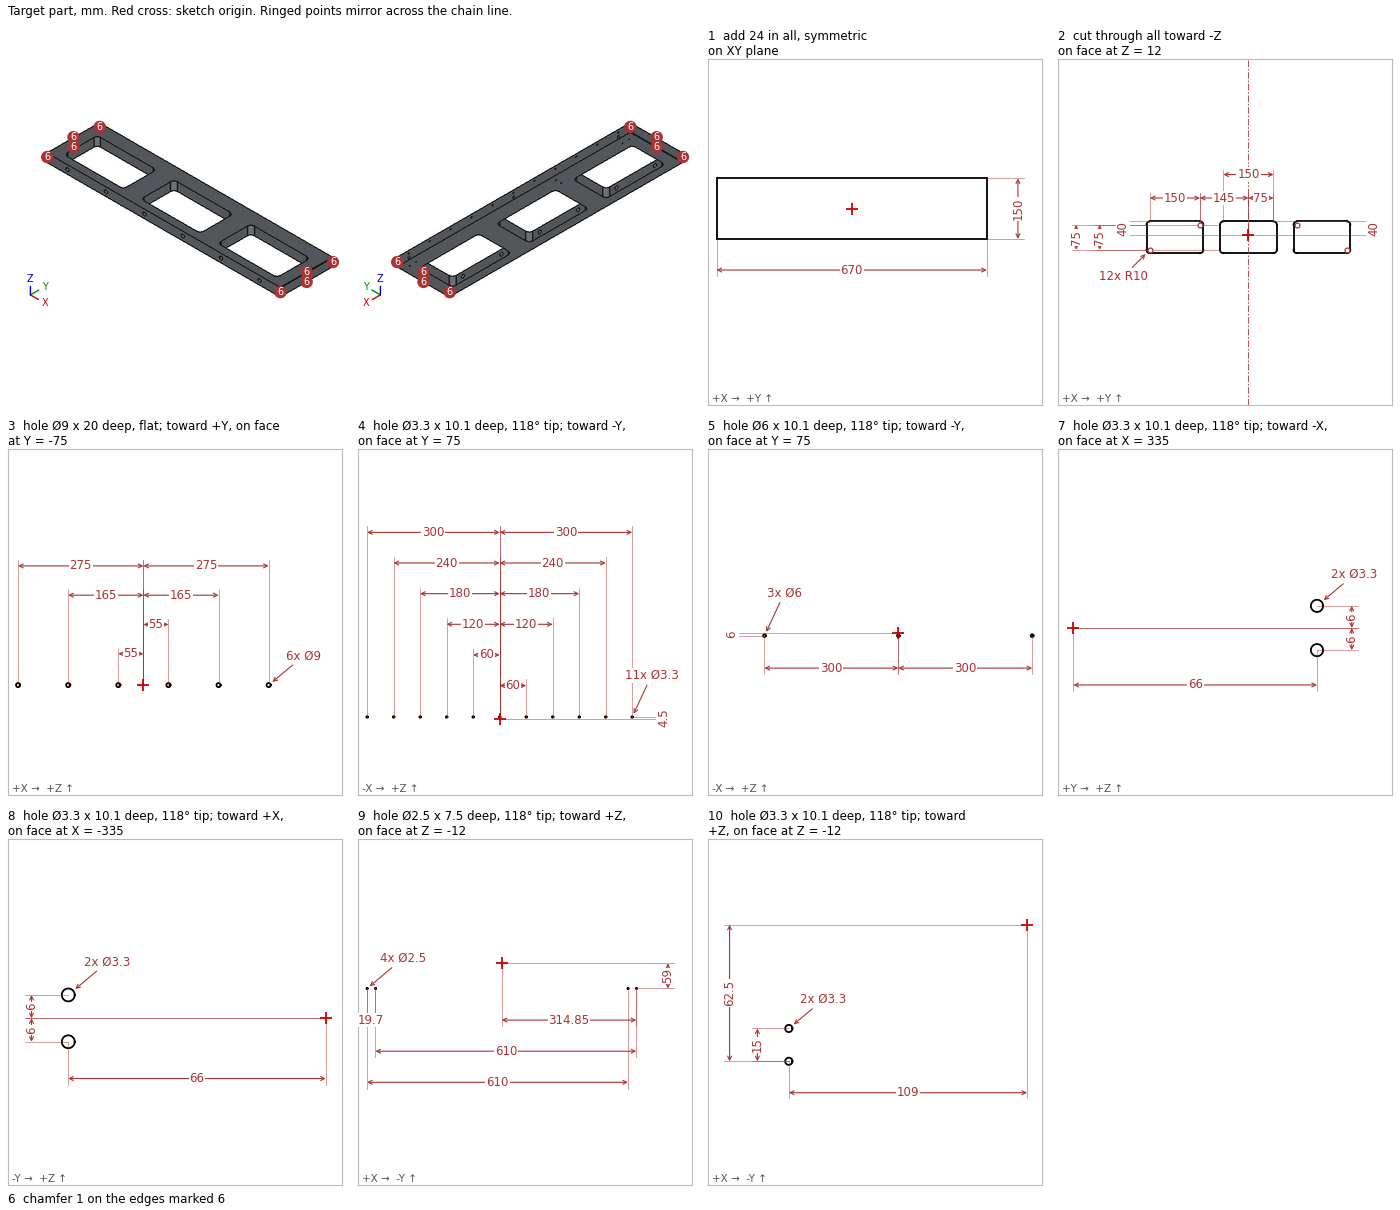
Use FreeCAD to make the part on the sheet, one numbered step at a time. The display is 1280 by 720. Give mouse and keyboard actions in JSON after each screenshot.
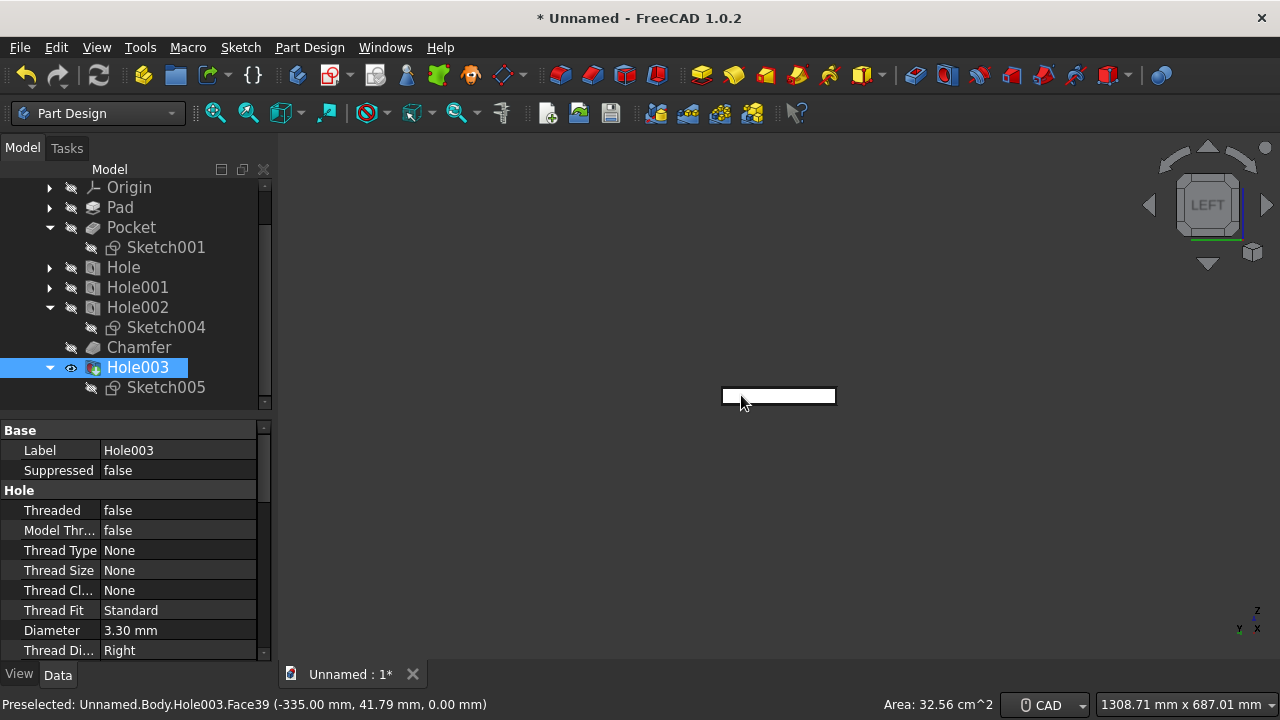
{"action": "left_click", "coordinate": [330, 76]}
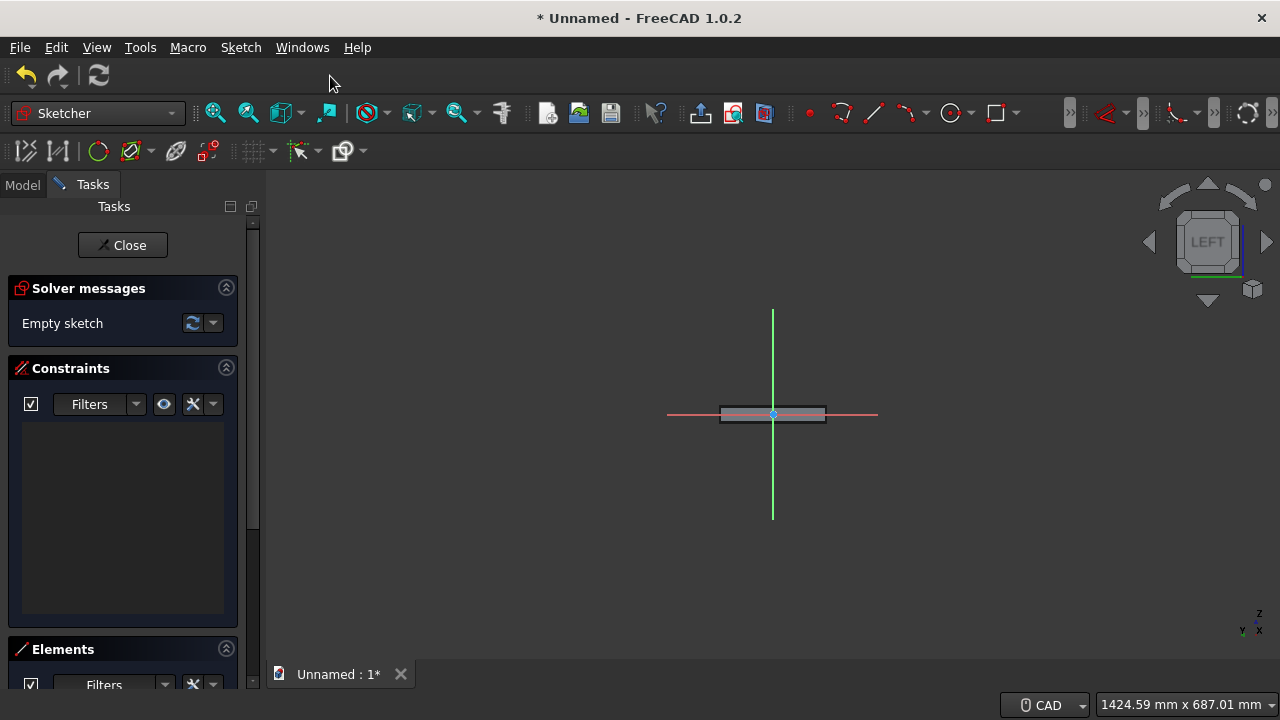
{"action": "scroll", "coordinate": [727, 414], "scroll_direction": "up", "scroll_amount": 15}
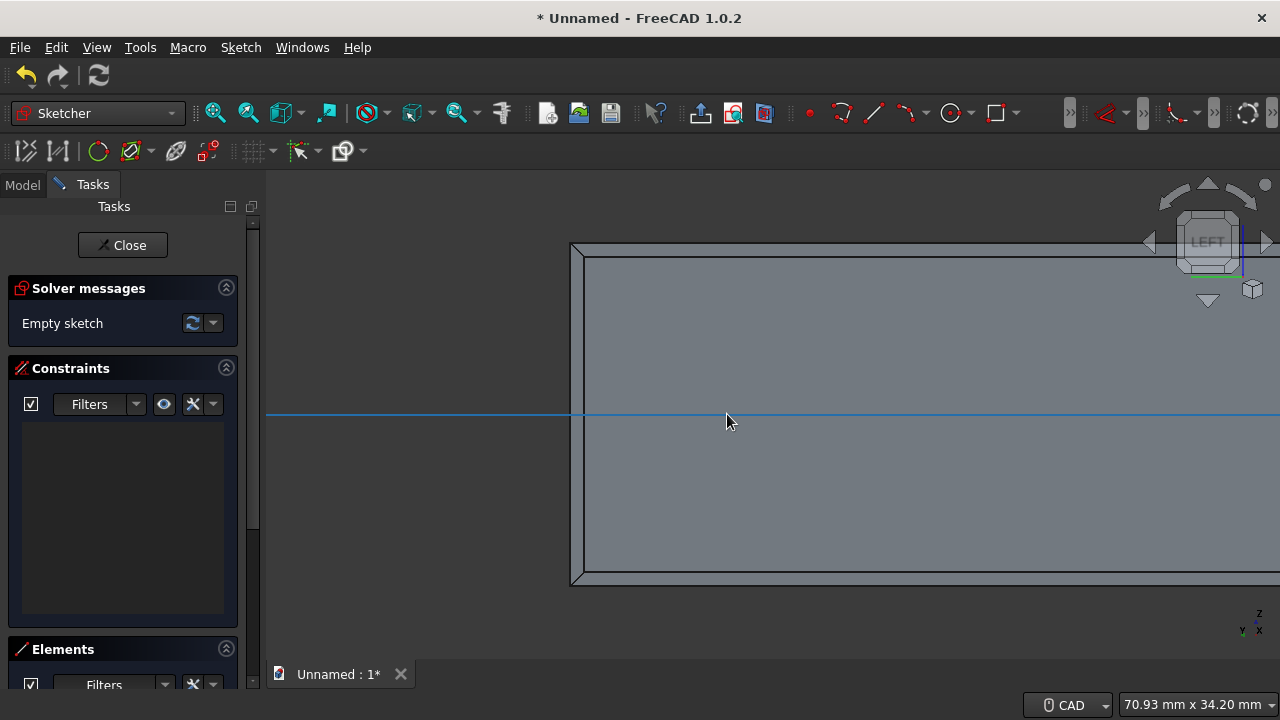
{"action": "scroll", "coordinate": [687, 414], "scroll_direction": "up", "scroll_amount": 2}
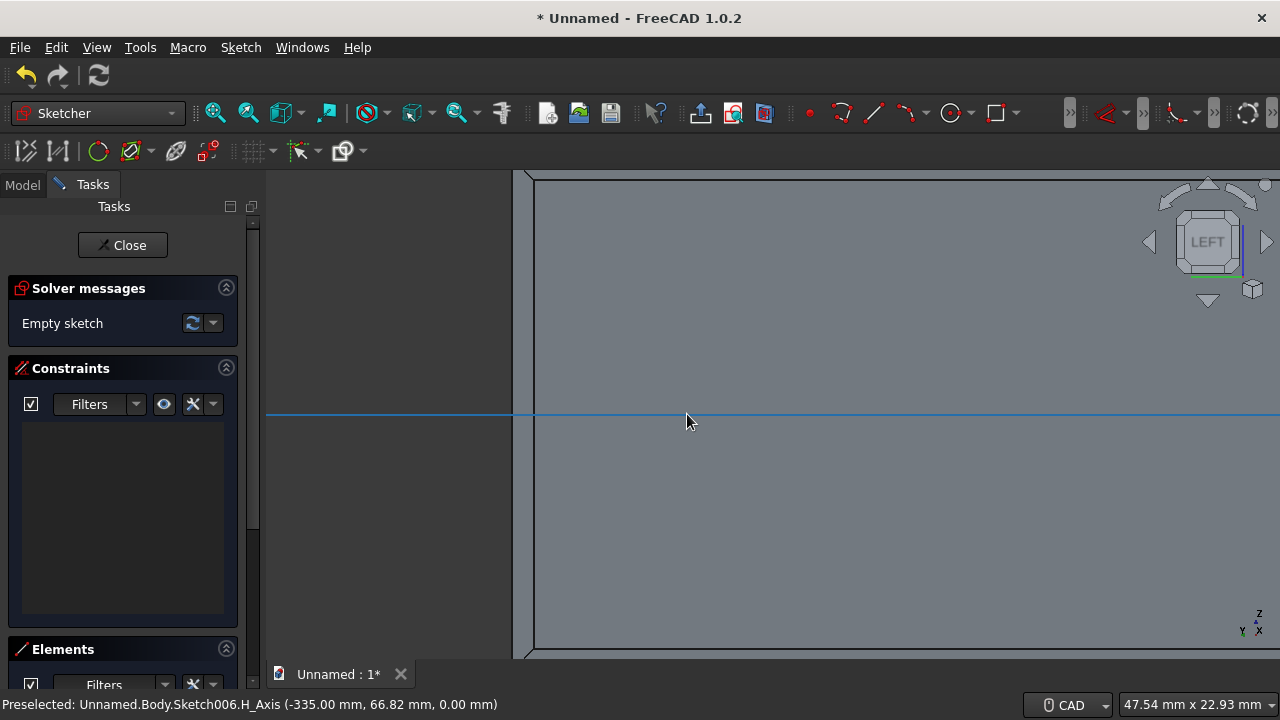
{"action": "left_click", "coordinate": [952, 114]}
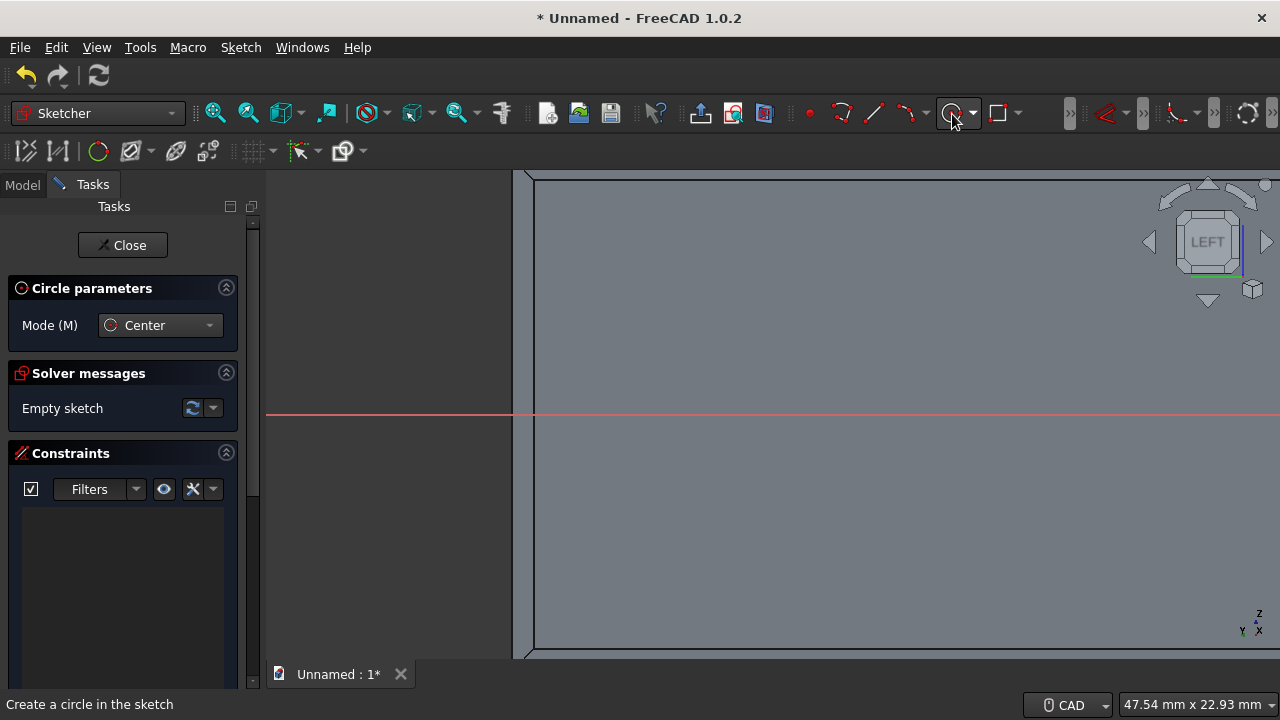
{"action": "left_click", "coordinate": [704, 542]}
{"action": "mouse_move", "coordinate": [729, 518]}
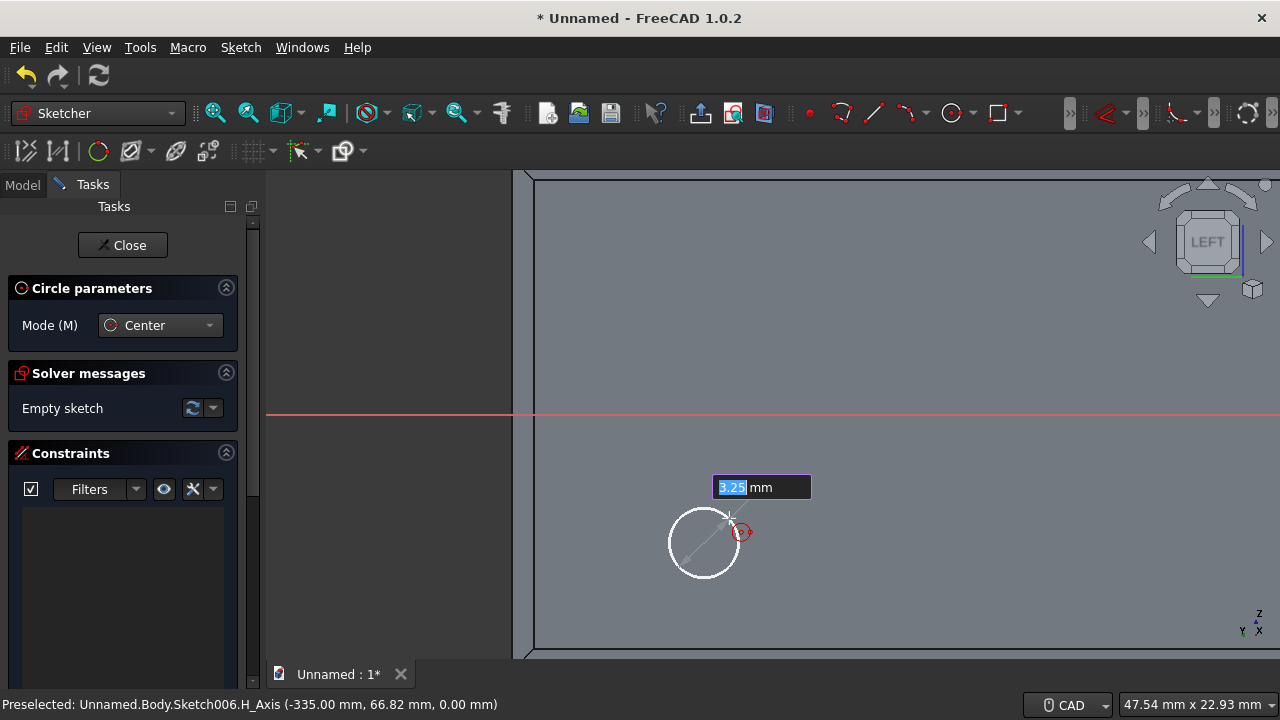
{"action": "type", "text": "3.3"}
{"action": "key", "text": "Return"}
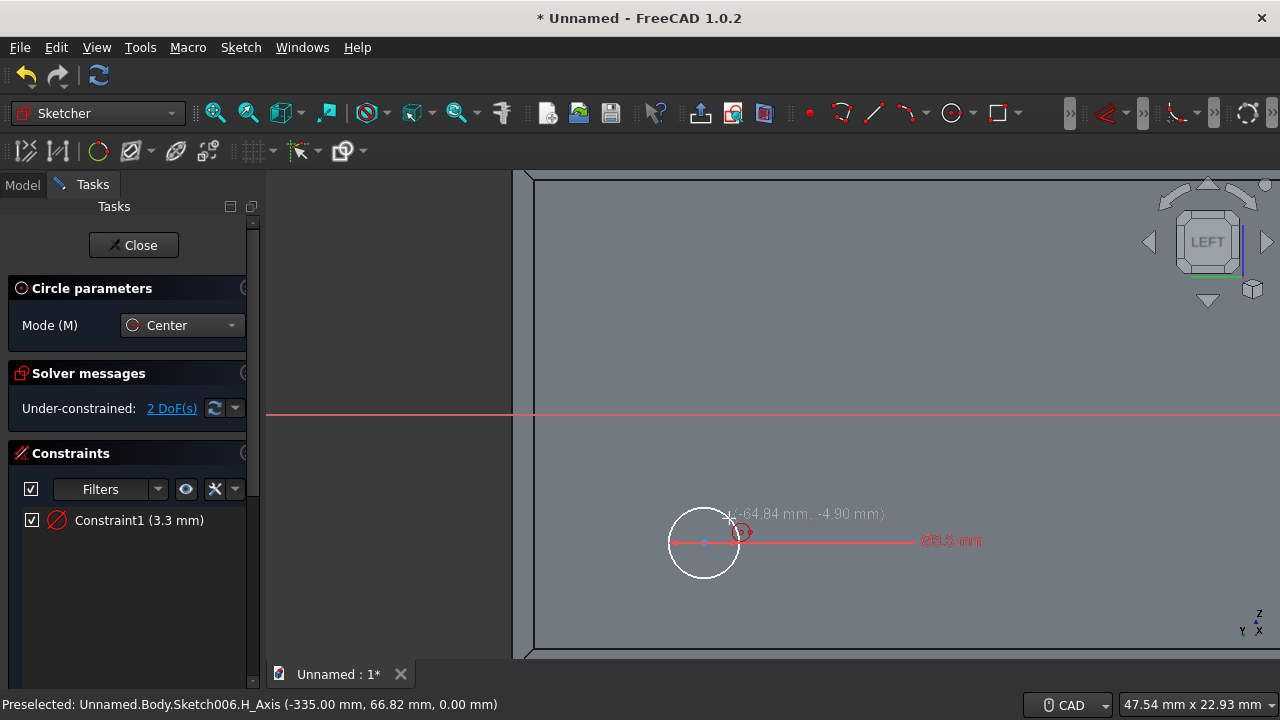
{"action": "left_click", "coordinate": [704, 287]}
{"action": "mouse_move", "coordinate": [729, 262]}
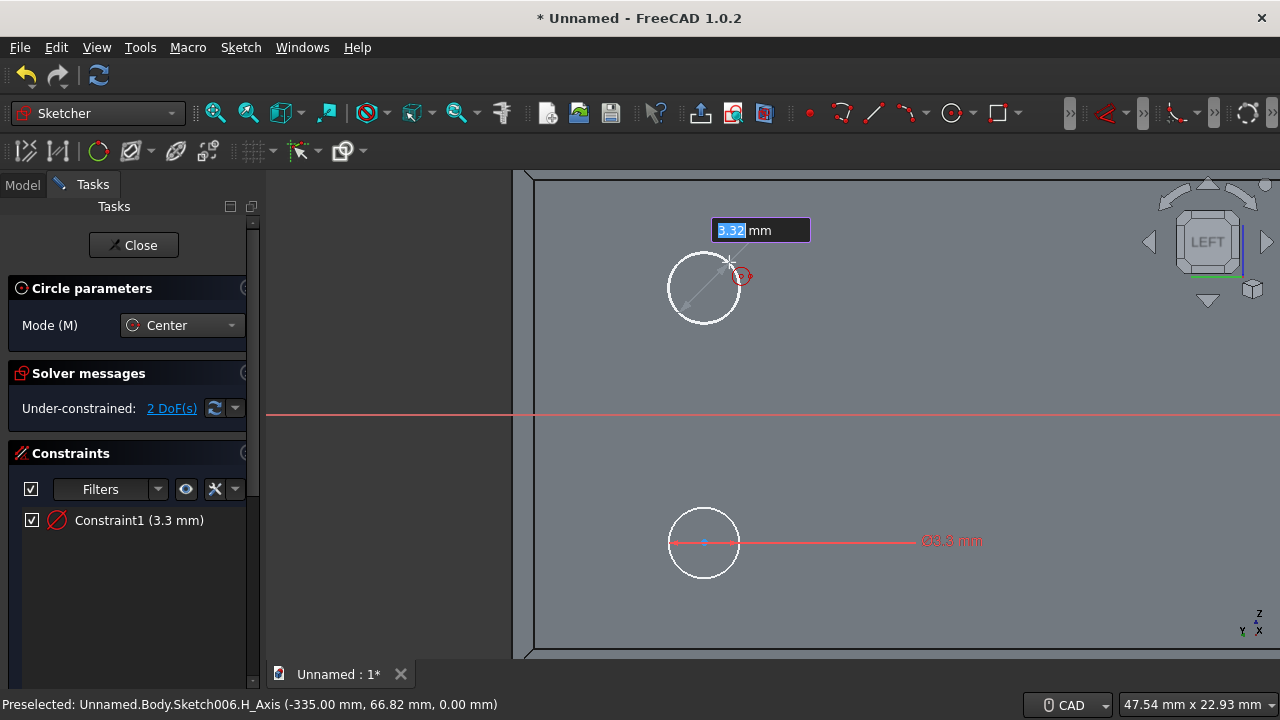
{"action": "type", "text": "3.3"}
{"action": "key", "text": "Return"}
{"action": "key", "text": "Escape"}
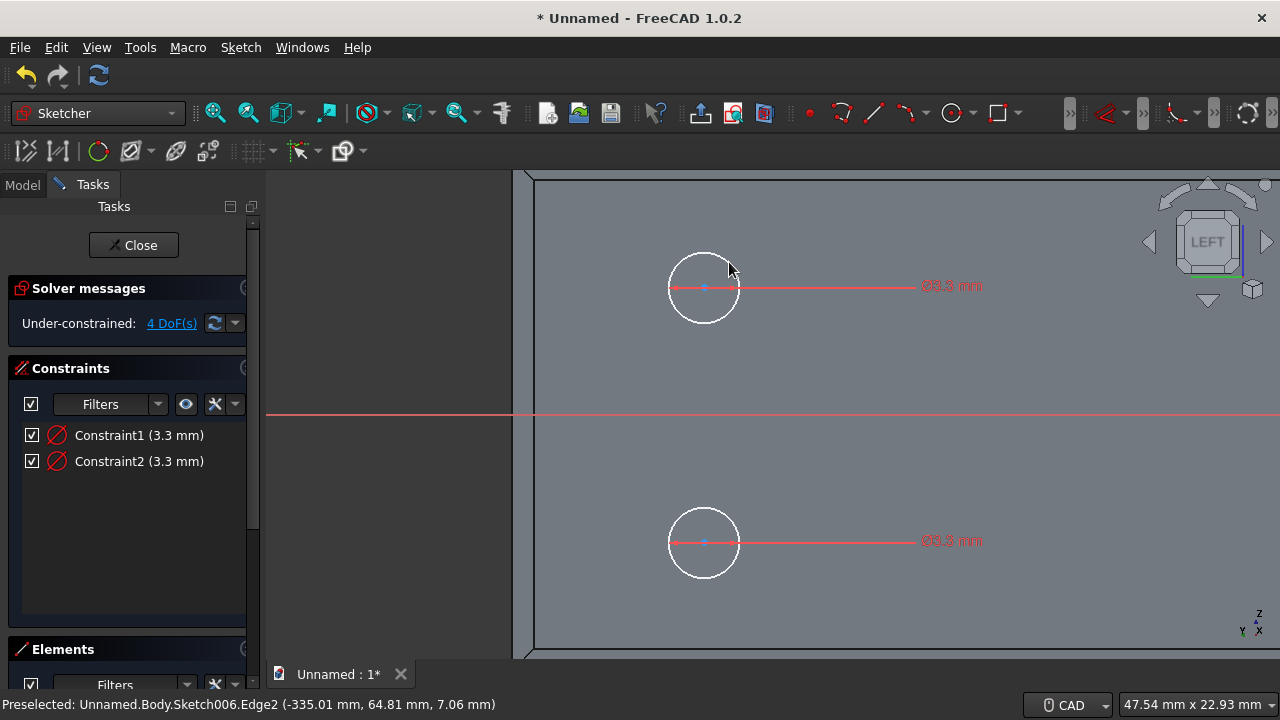
{"action": "left_click", "coordinate": [704, 543]}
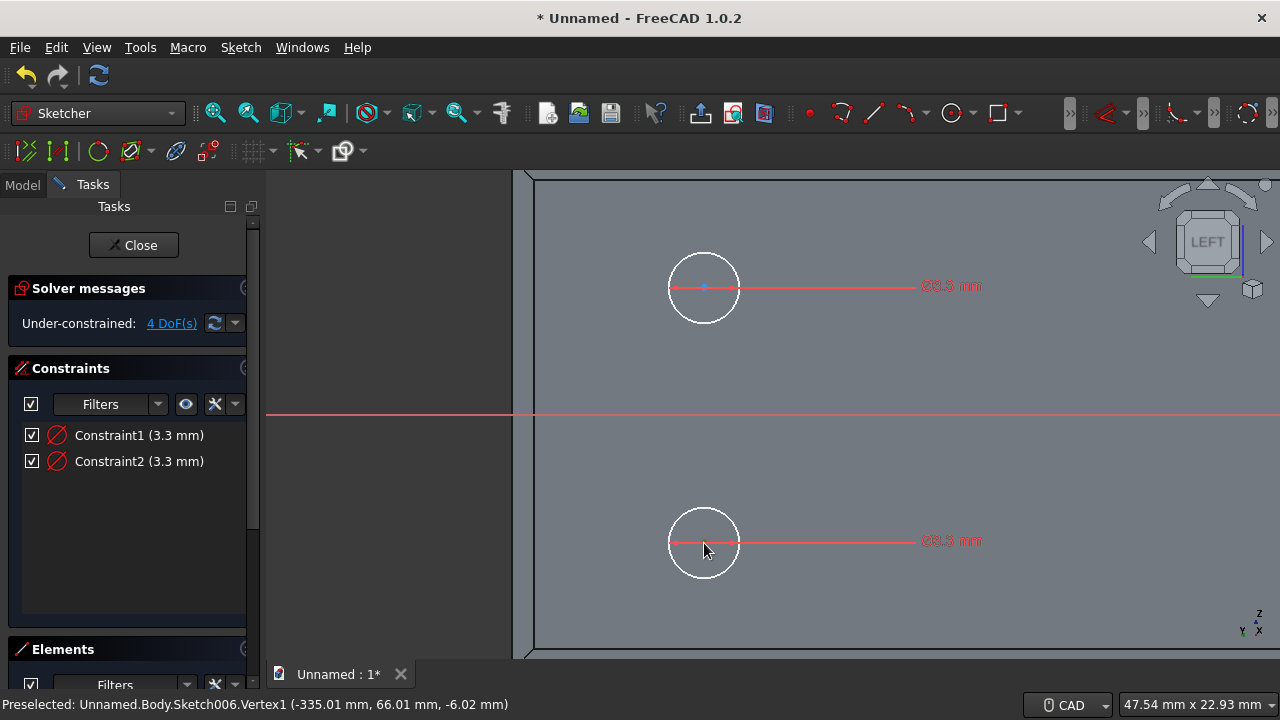
{"action": "left_click", "coordinate": [704, 288]}